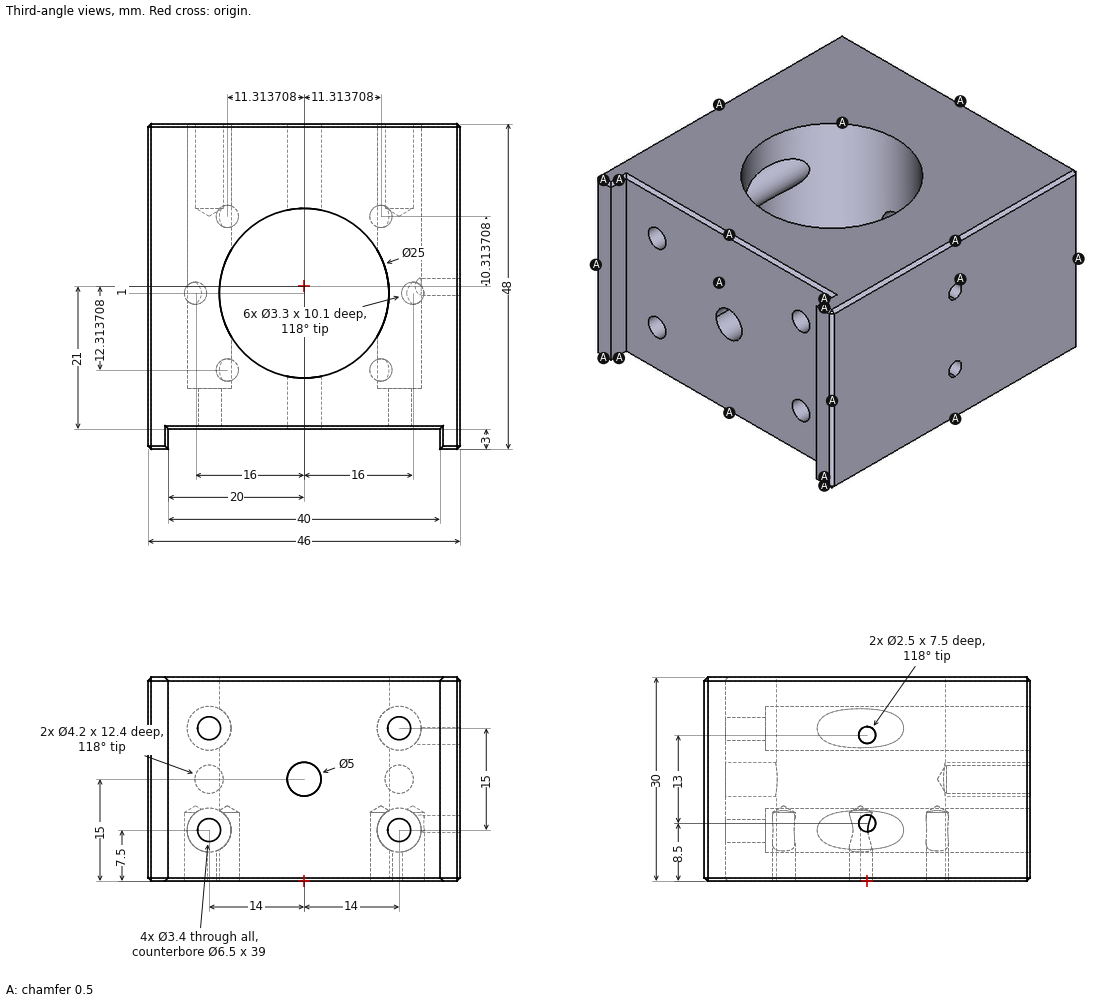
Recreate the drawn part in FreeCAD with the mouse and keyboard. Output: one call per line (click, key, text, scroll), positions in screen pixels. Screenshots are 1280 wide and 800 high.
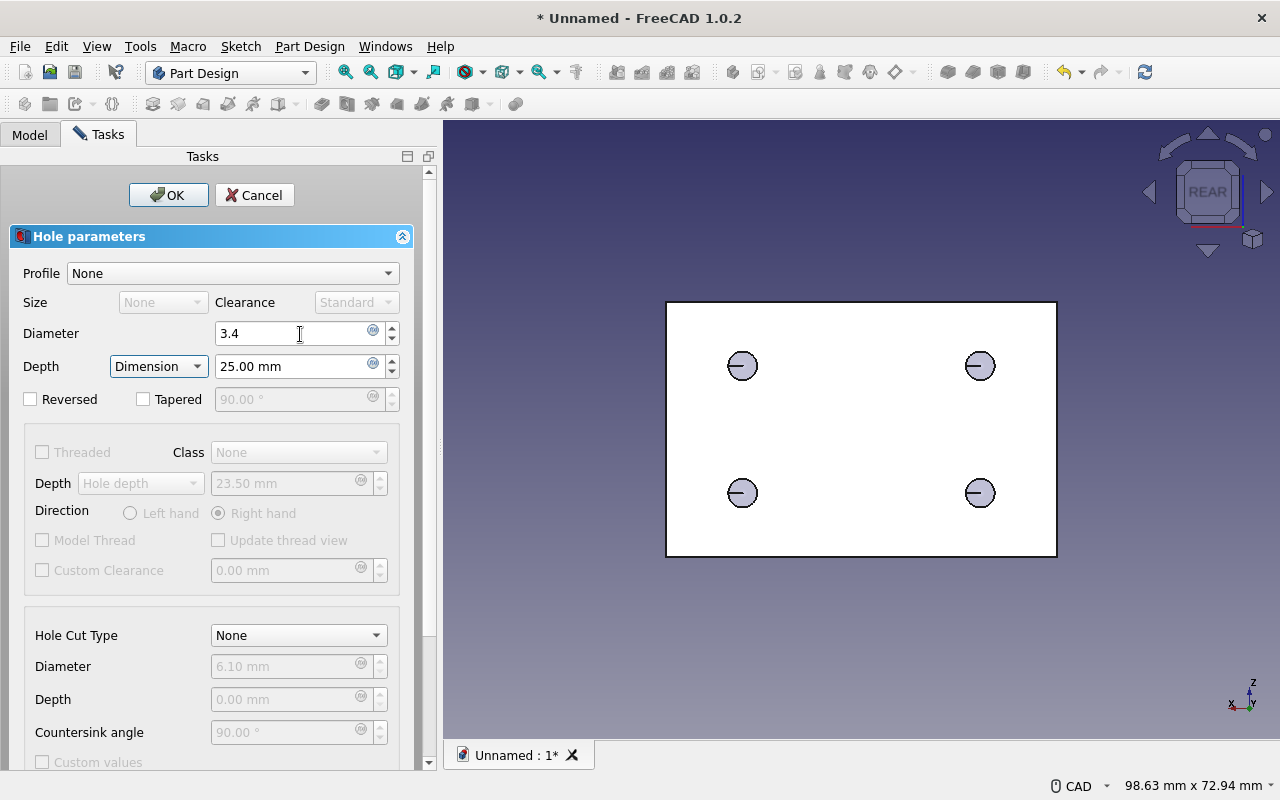
click(160, 366)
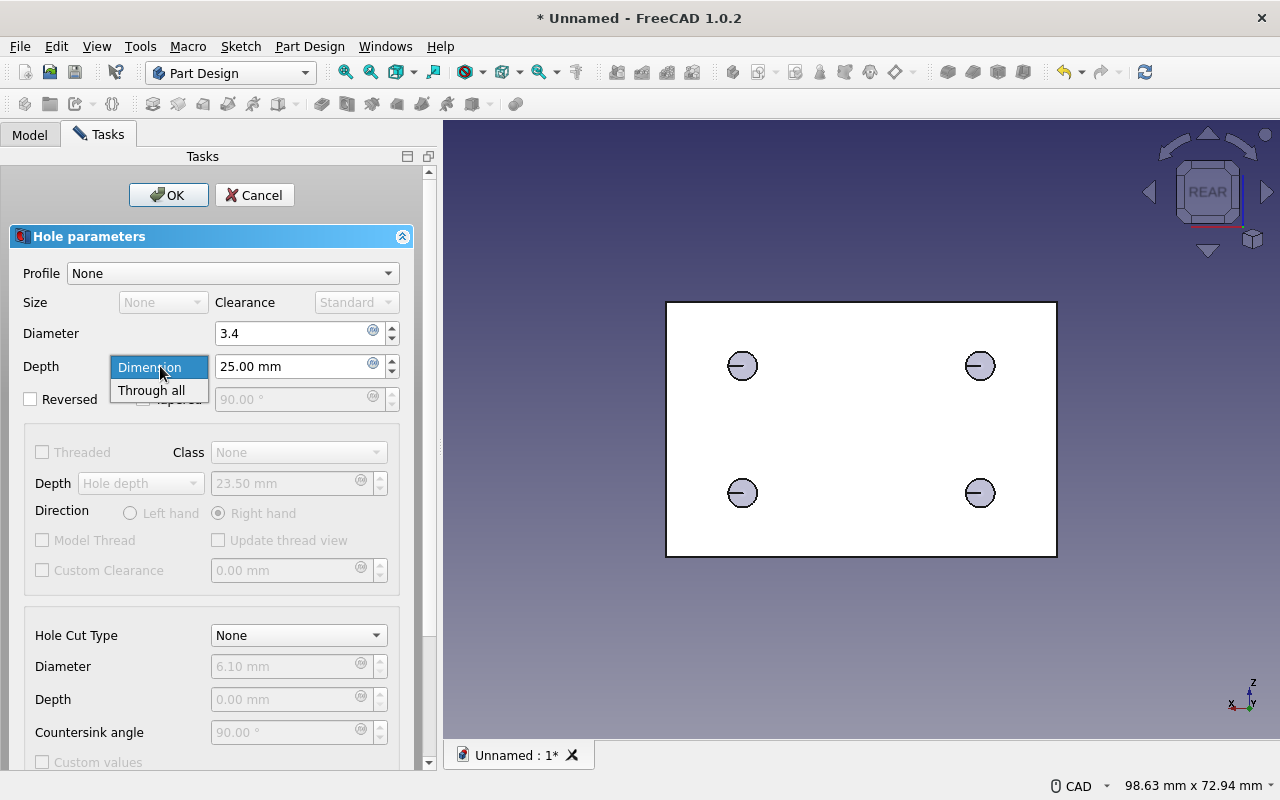
click(158, 390)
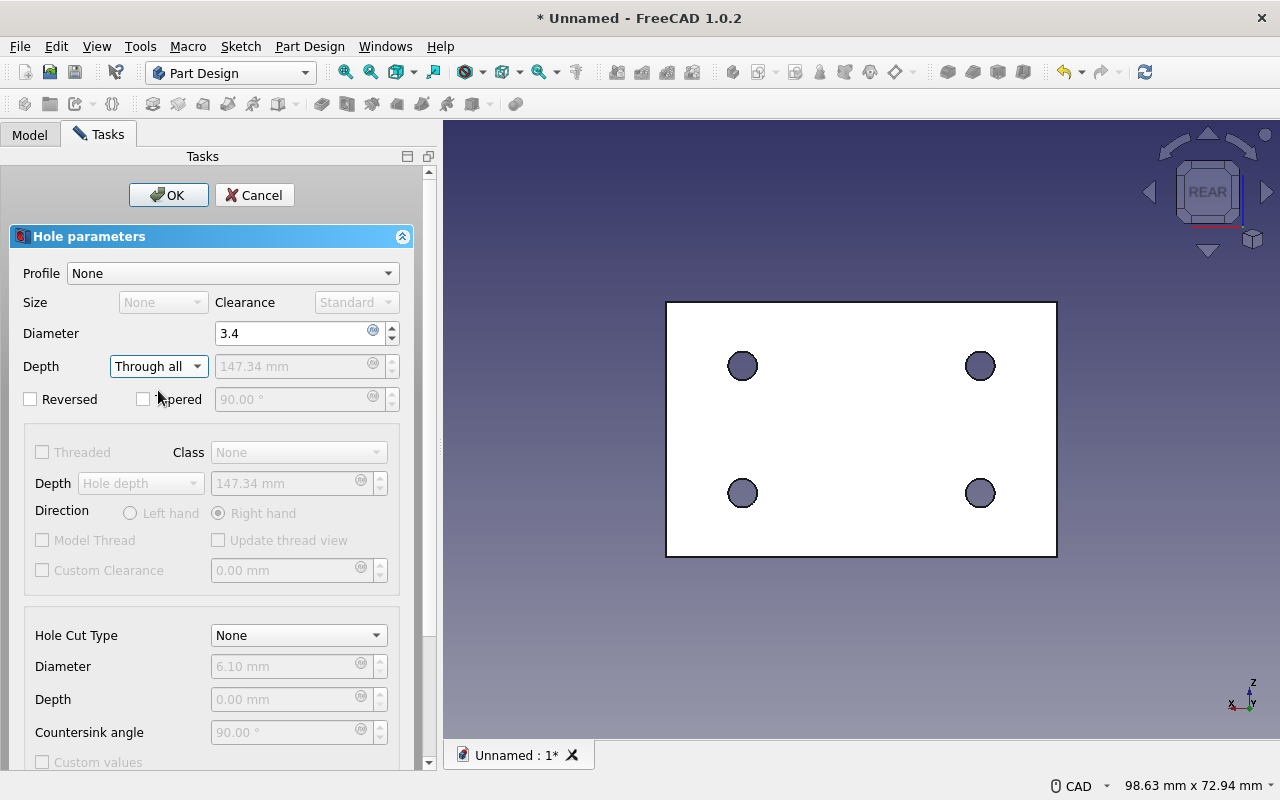
click(300, 636)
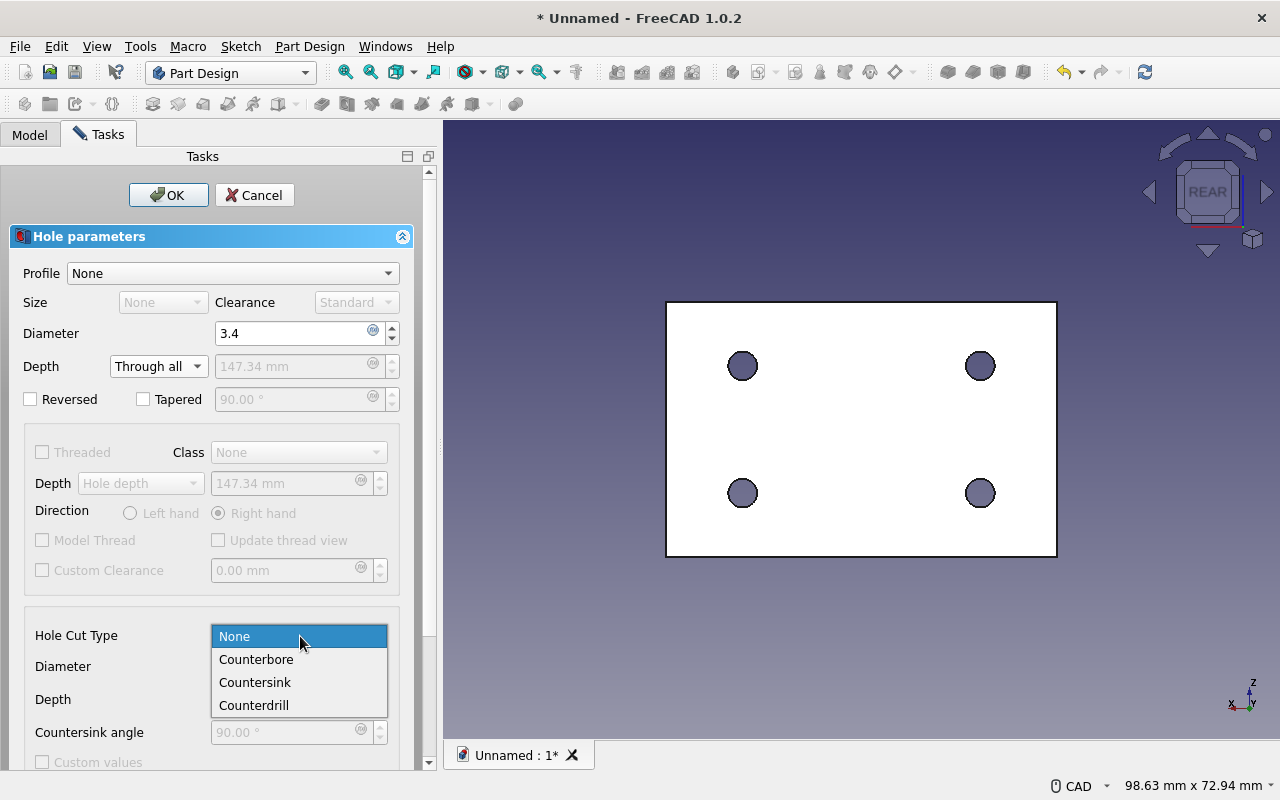
click(298, 660)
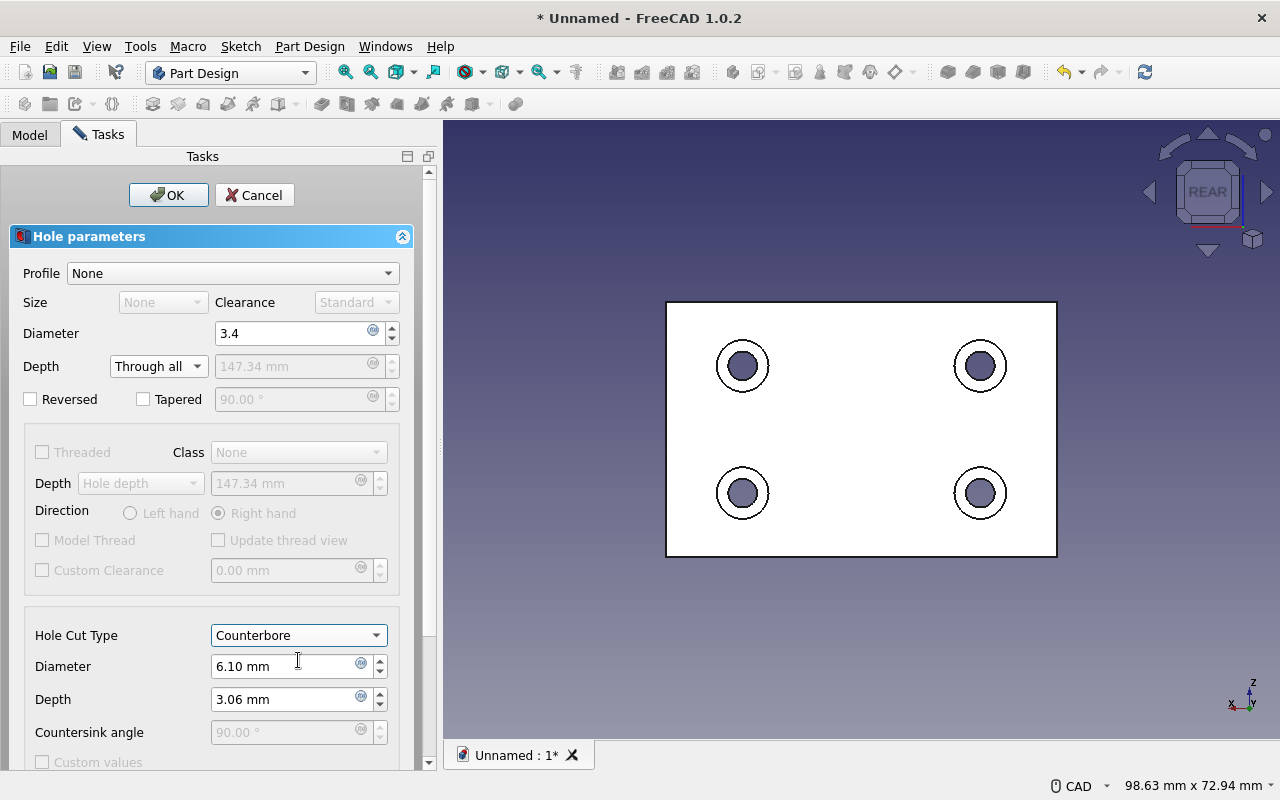
triple_click(292, 666)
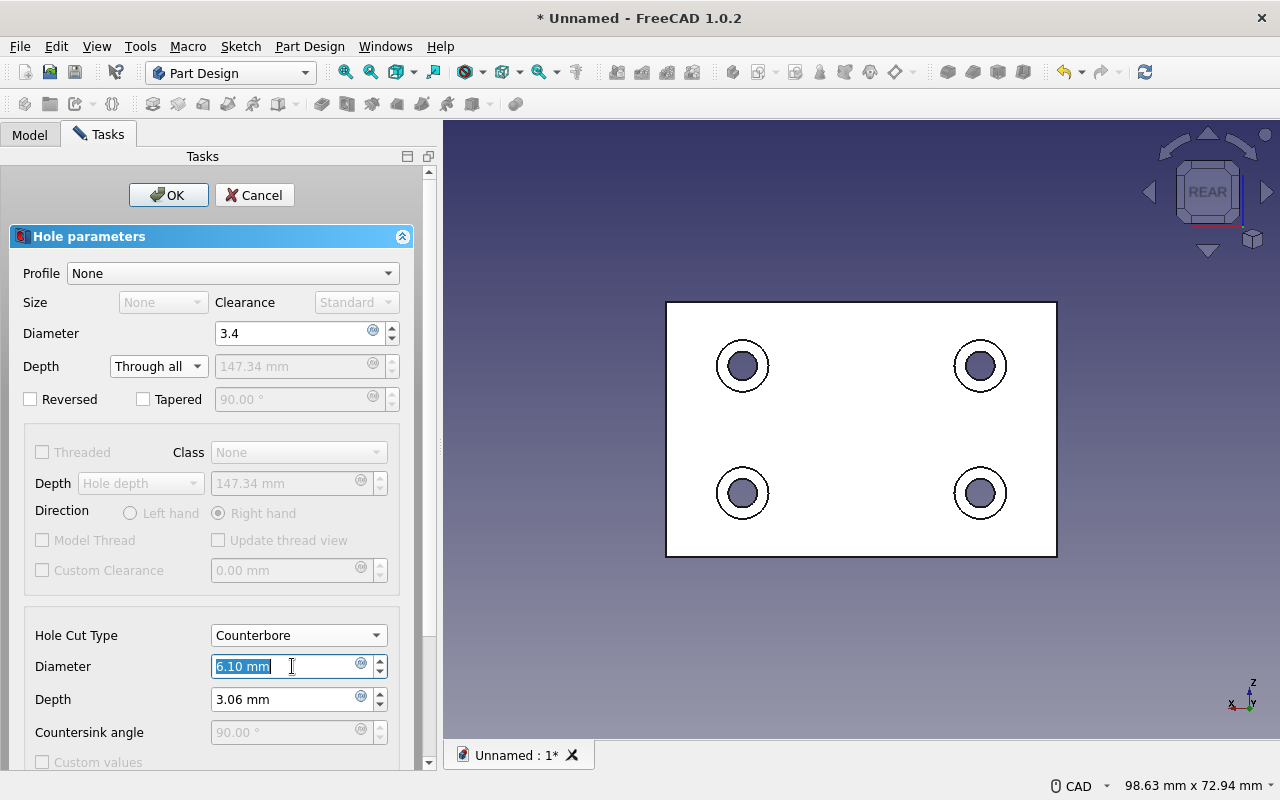
text(6.5)
key(Tab)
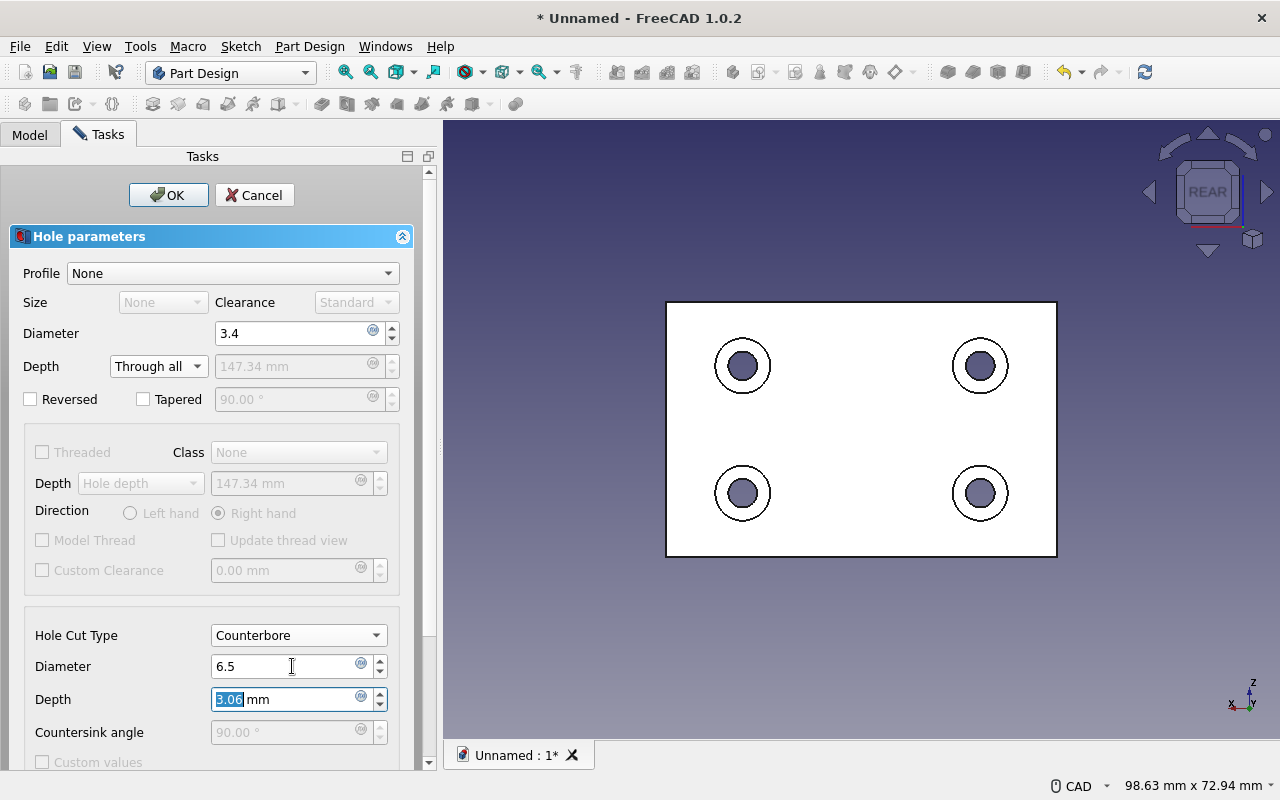
text(39)
key(Tab)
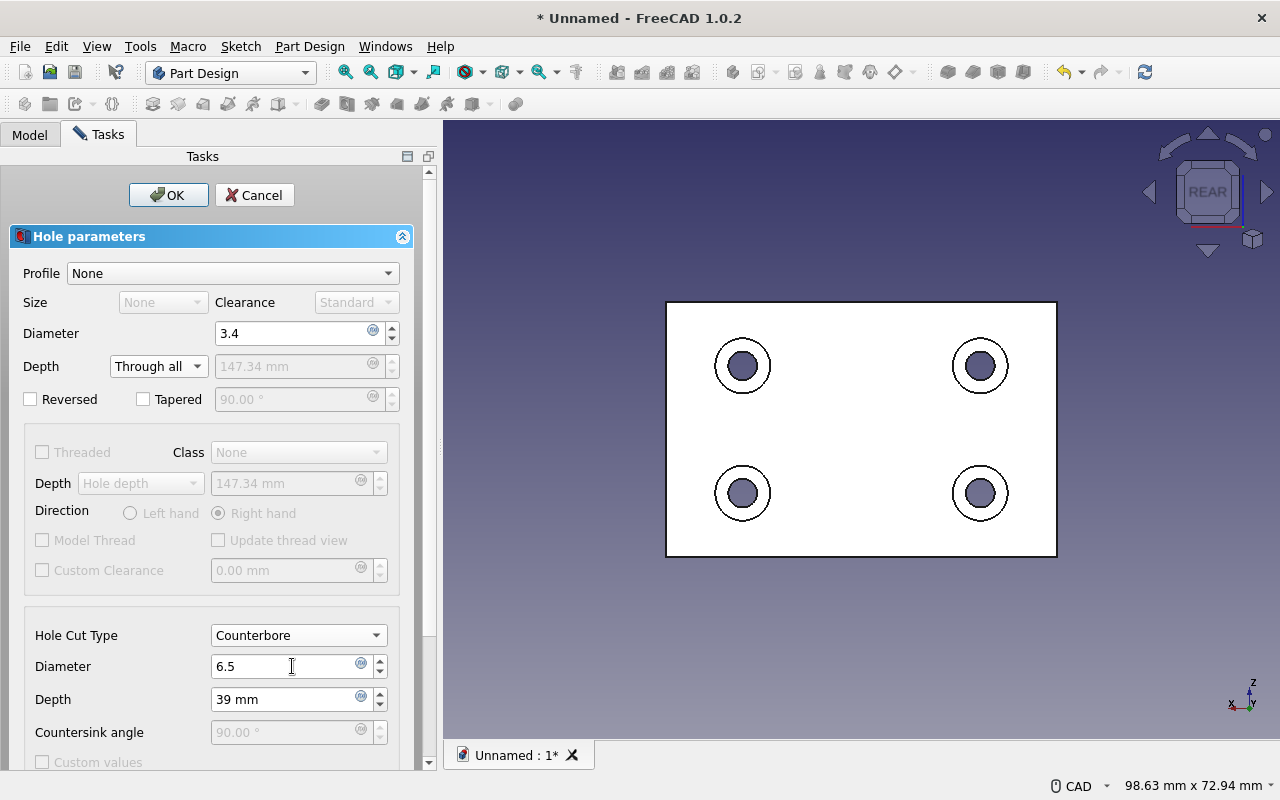
click(169, 195)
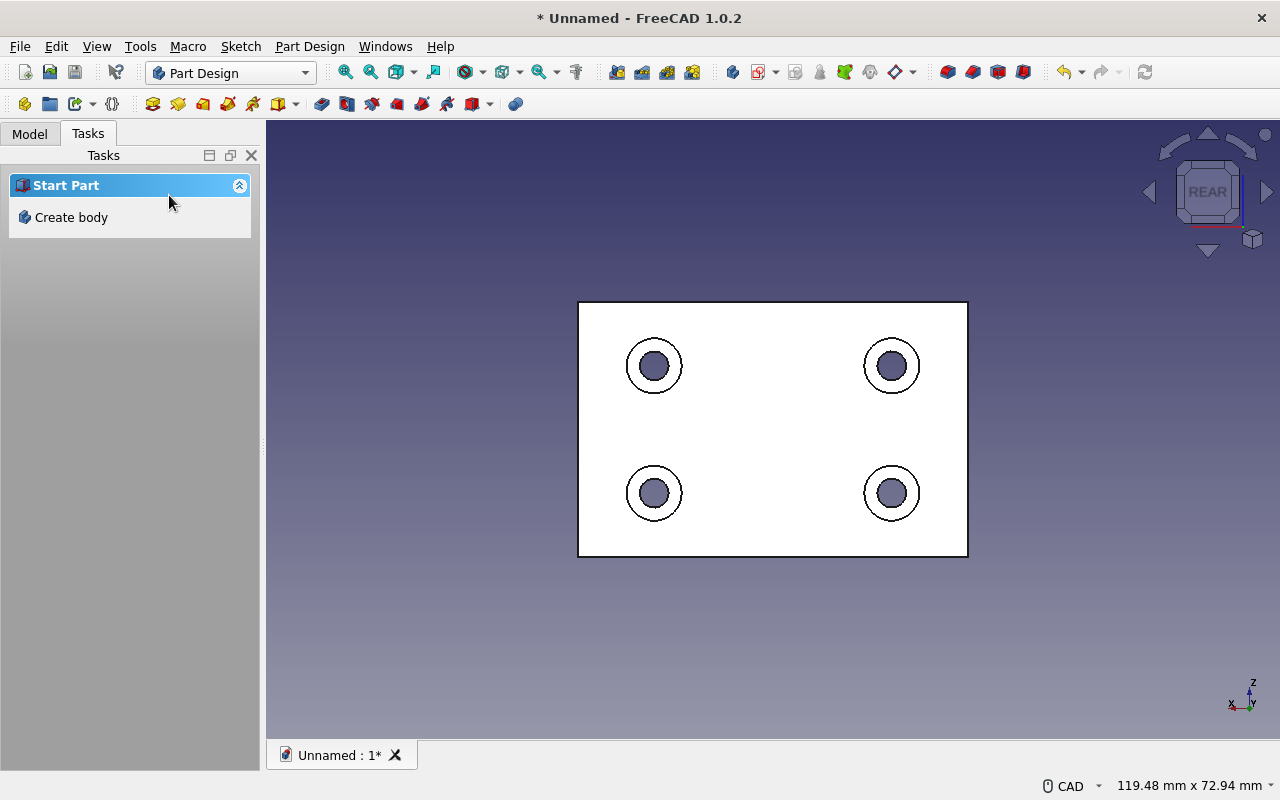
click(346, 72)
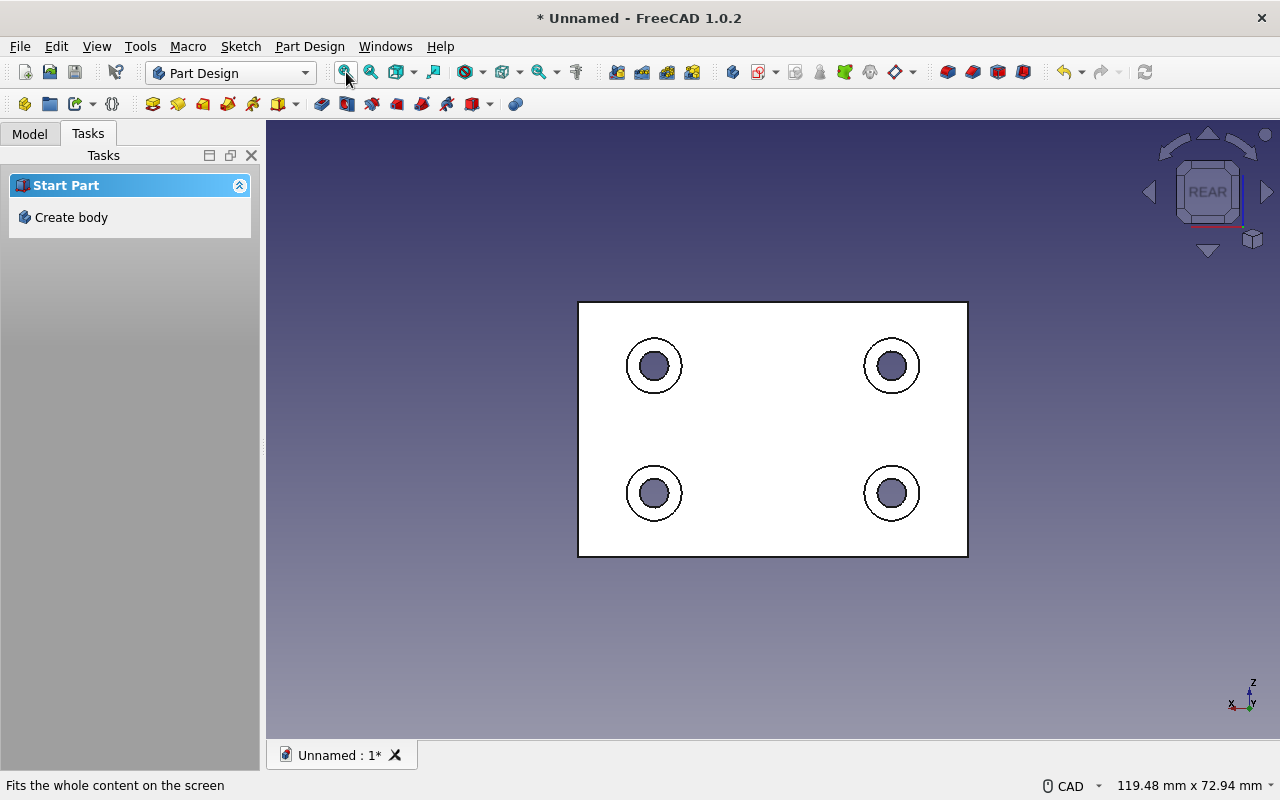
key(0)